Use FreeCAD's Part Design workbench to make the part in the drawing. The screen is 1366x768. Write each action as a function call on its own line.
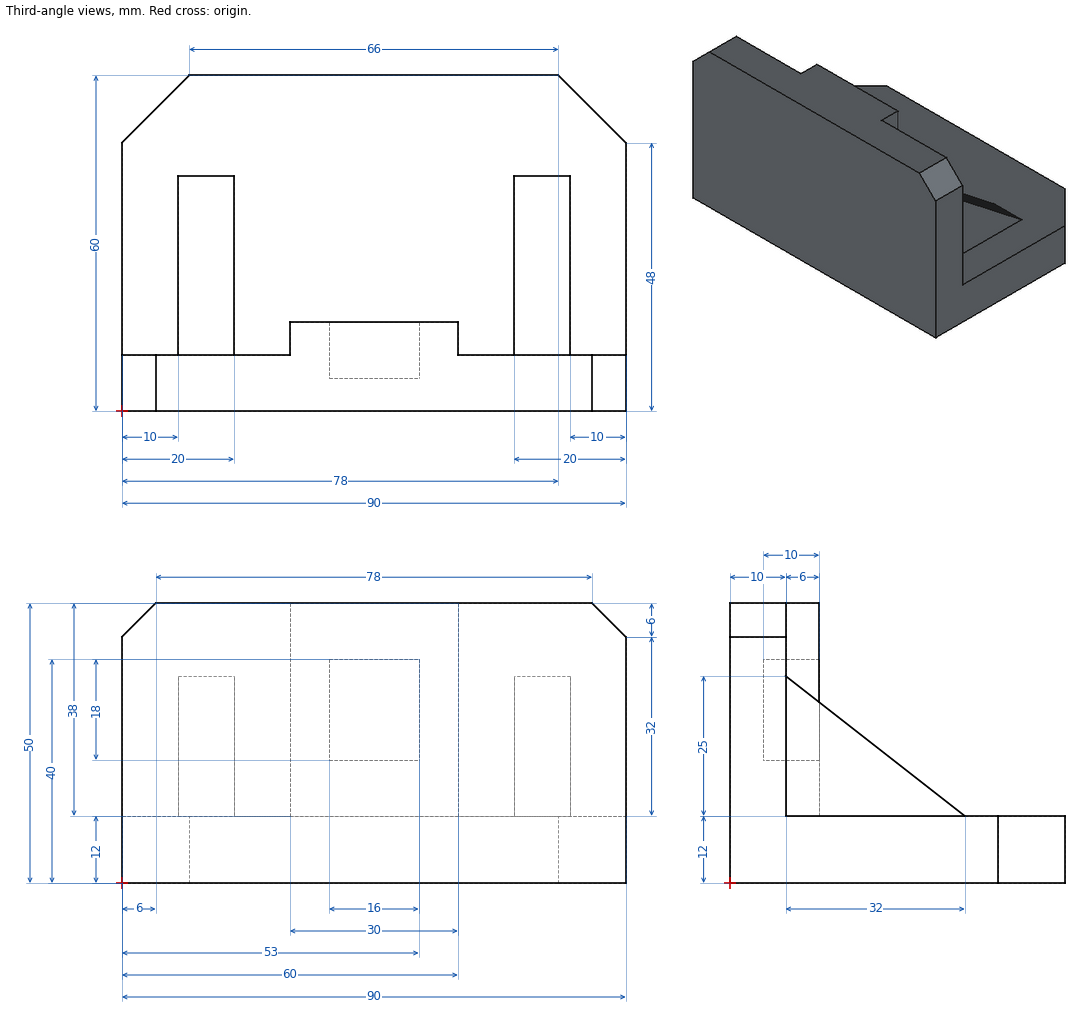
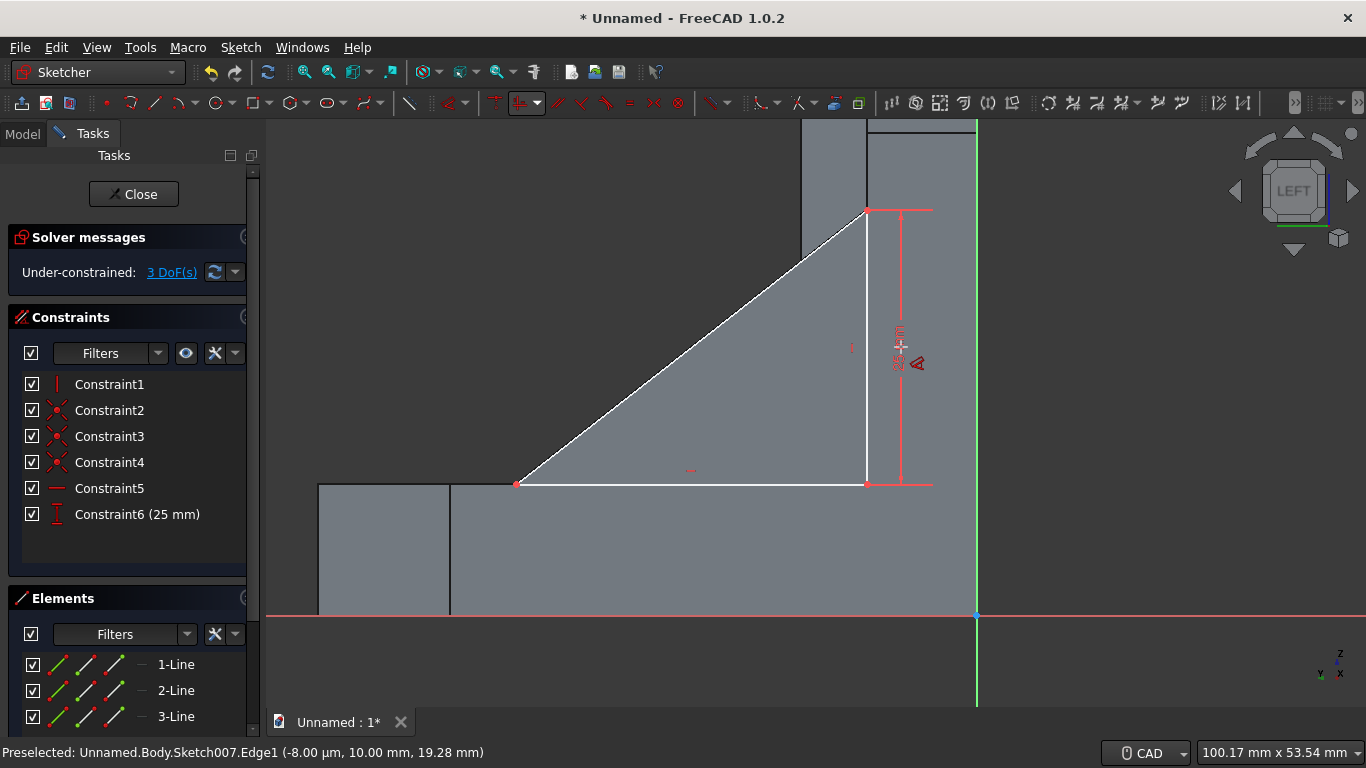
click(621, 485)
click(692, 519)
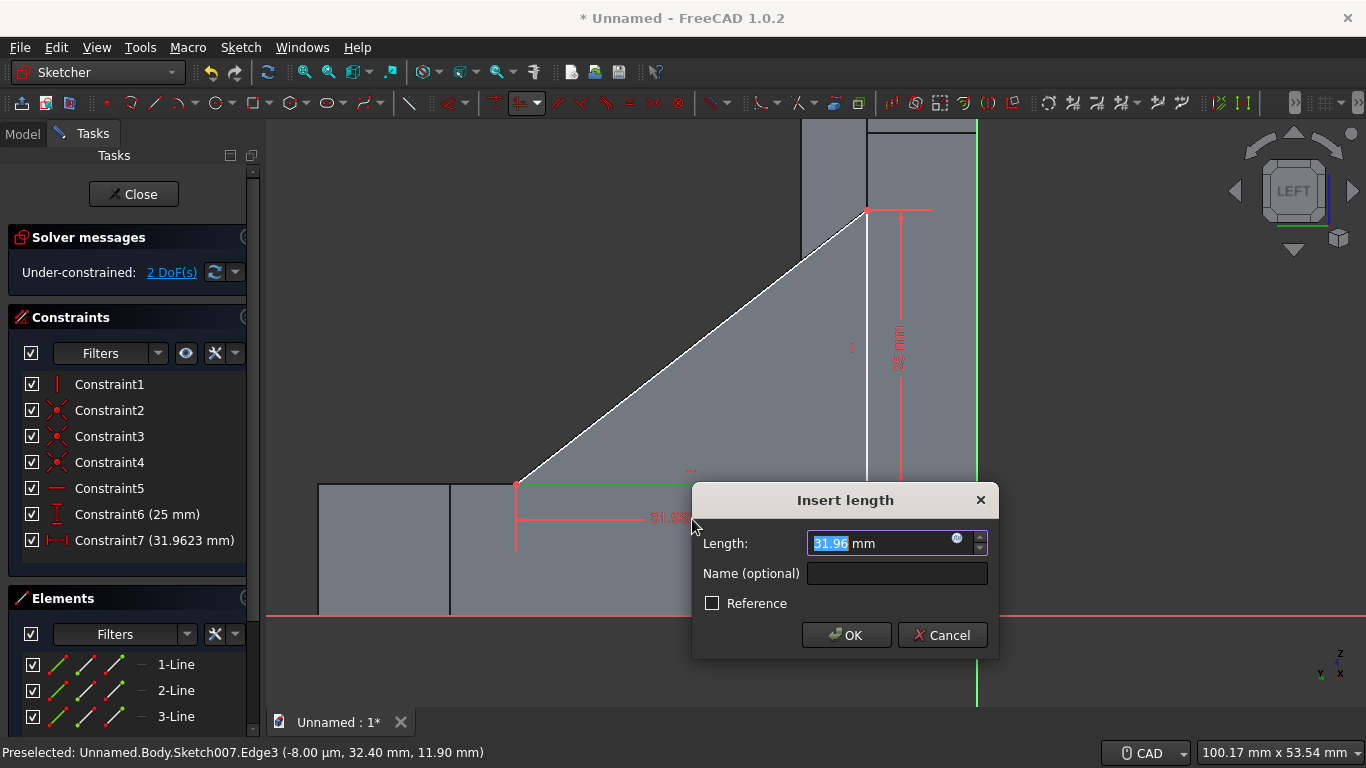
text(32)
key(Return)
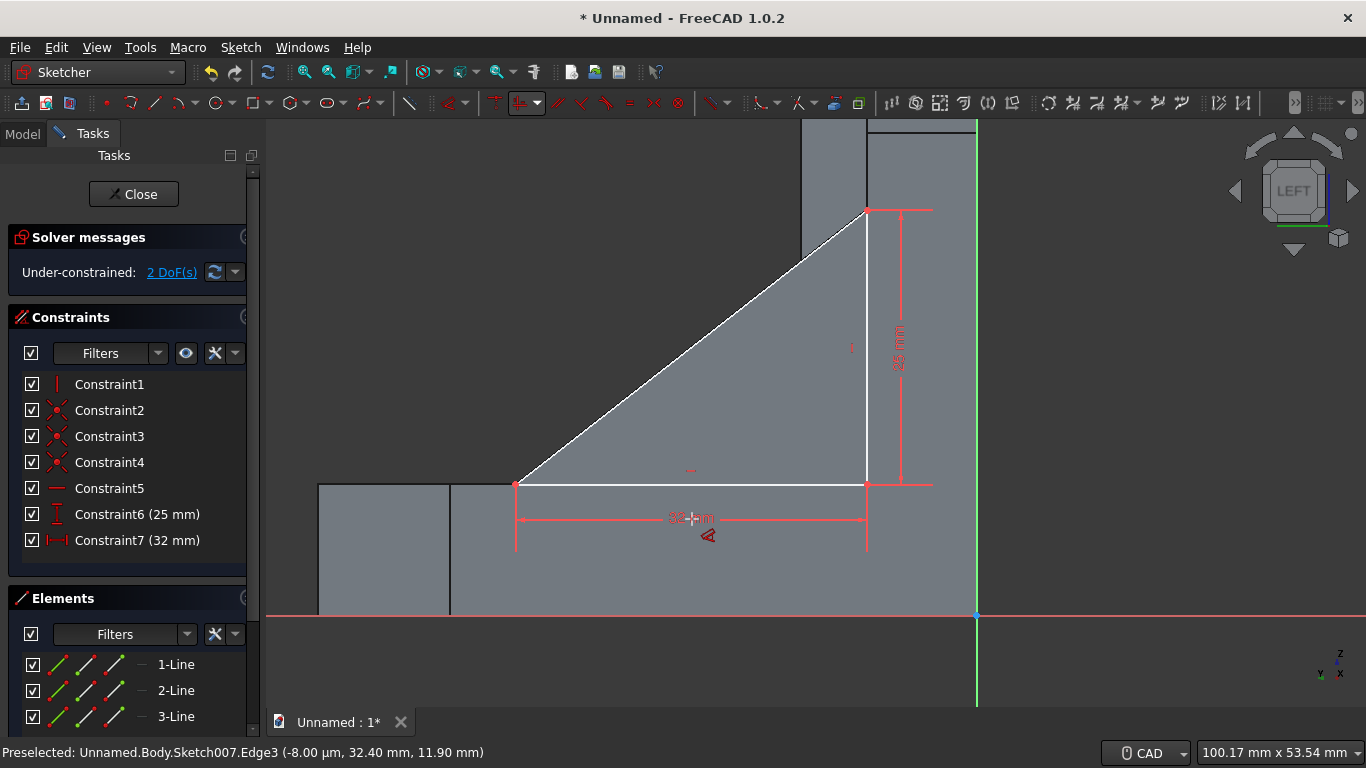
click(867, 485)
click(922, 650)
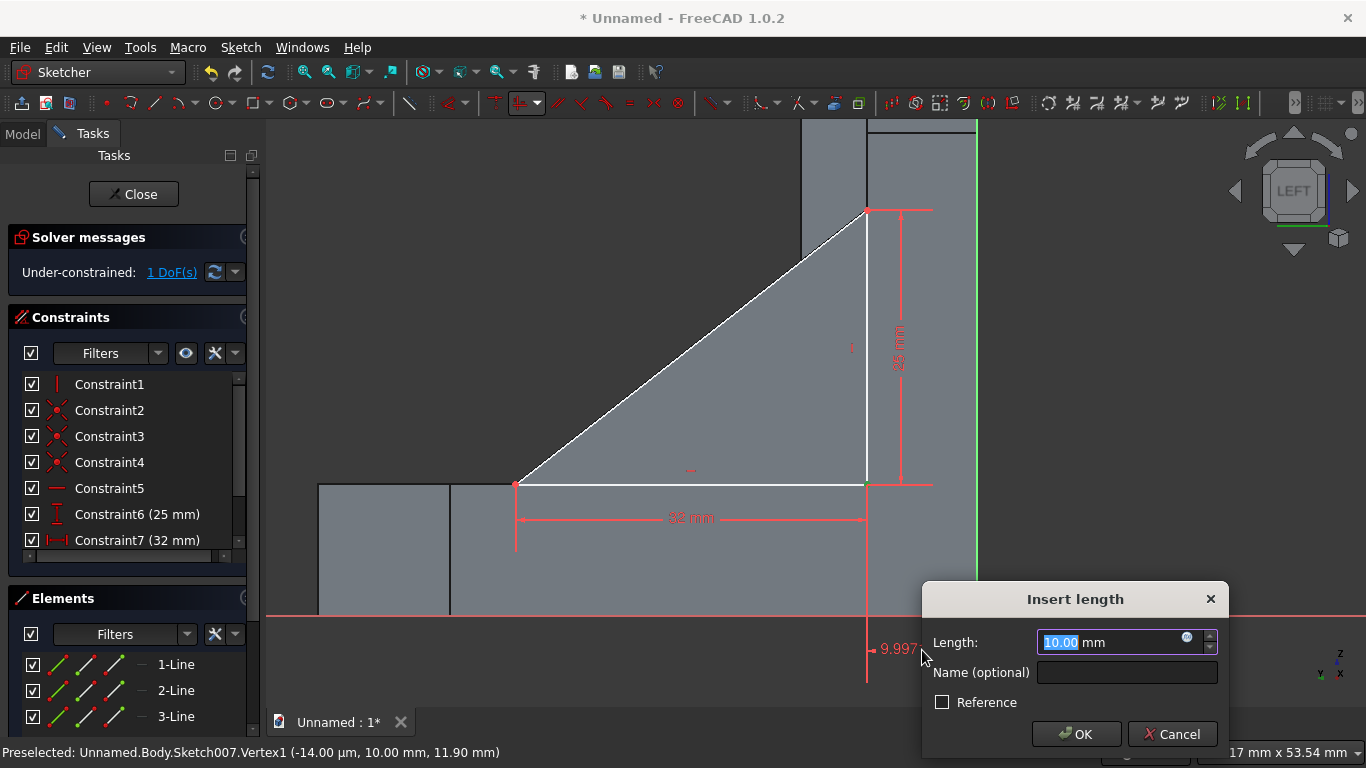
text(10)
key(Return)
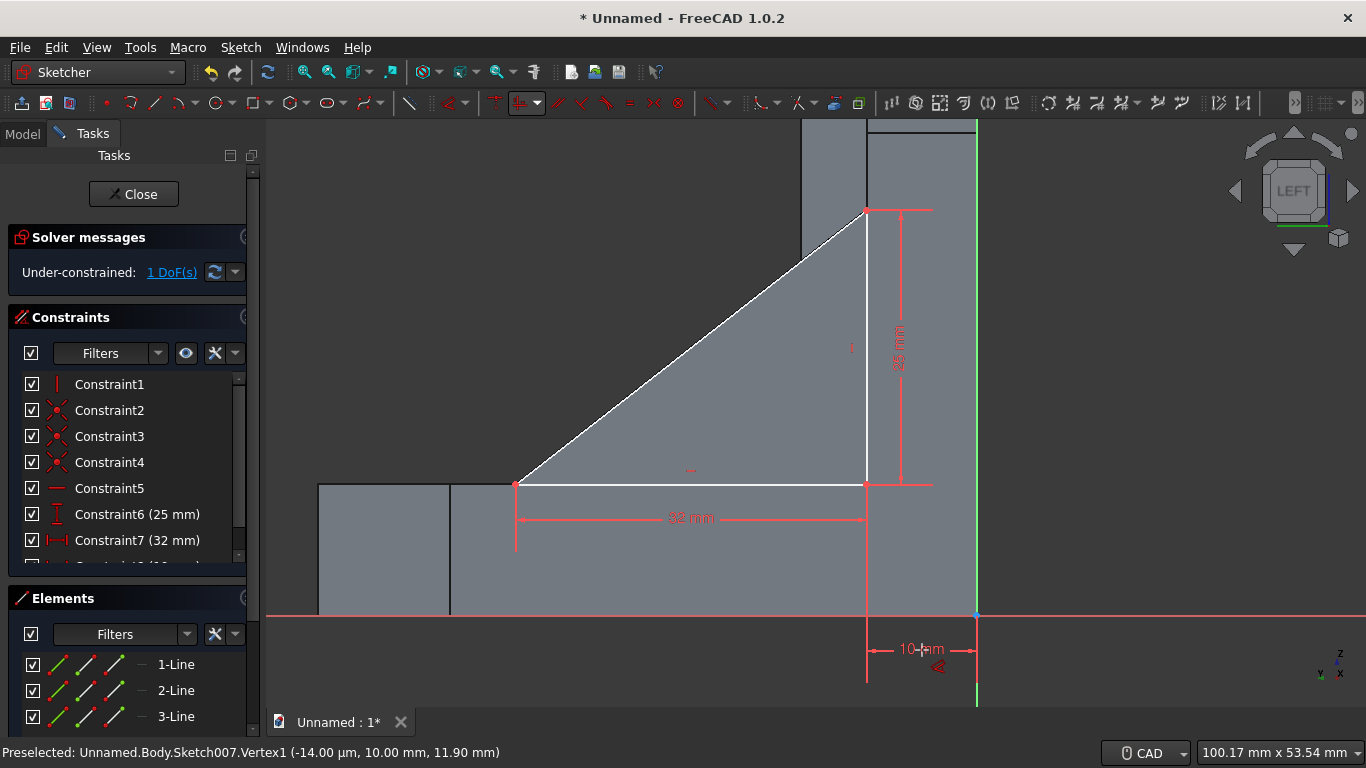
click(867, 485)
click(1011, 550)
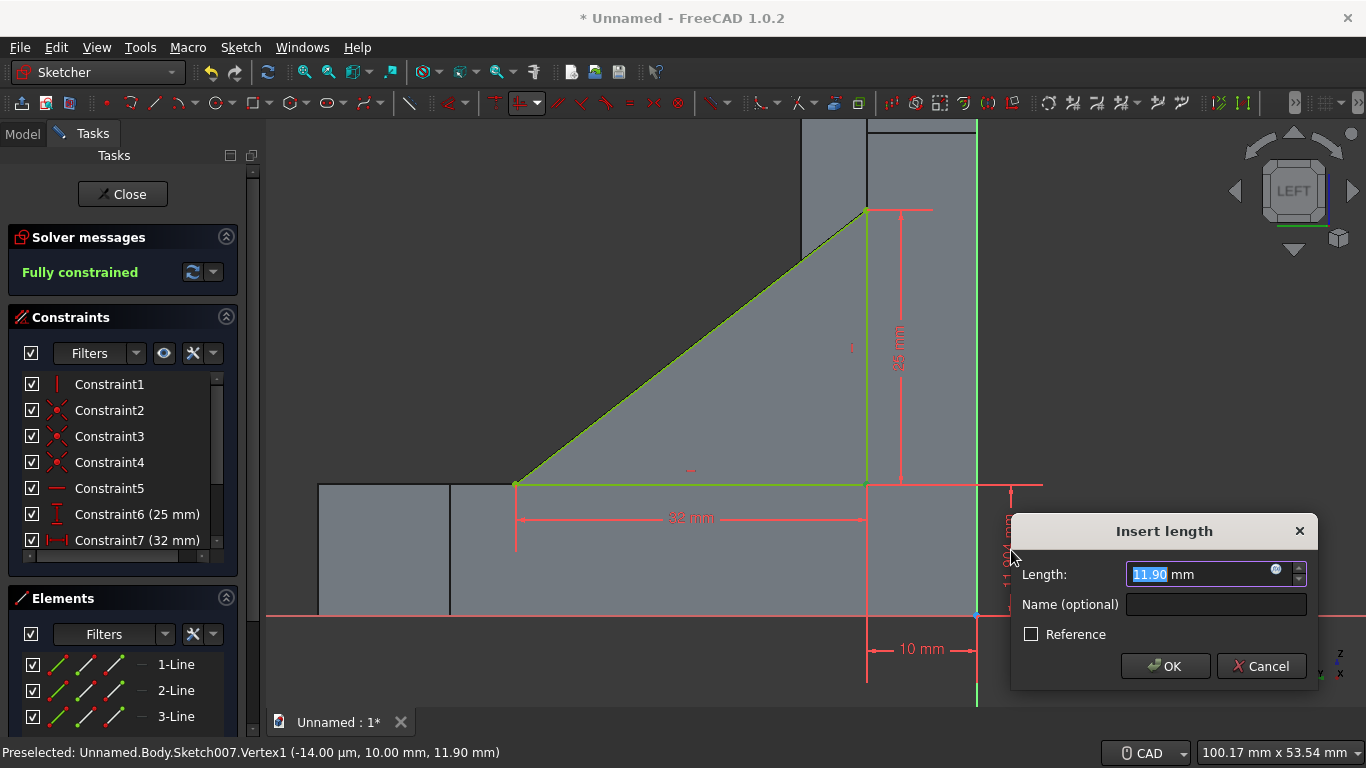
text(12)
key(Return)
key(Escape)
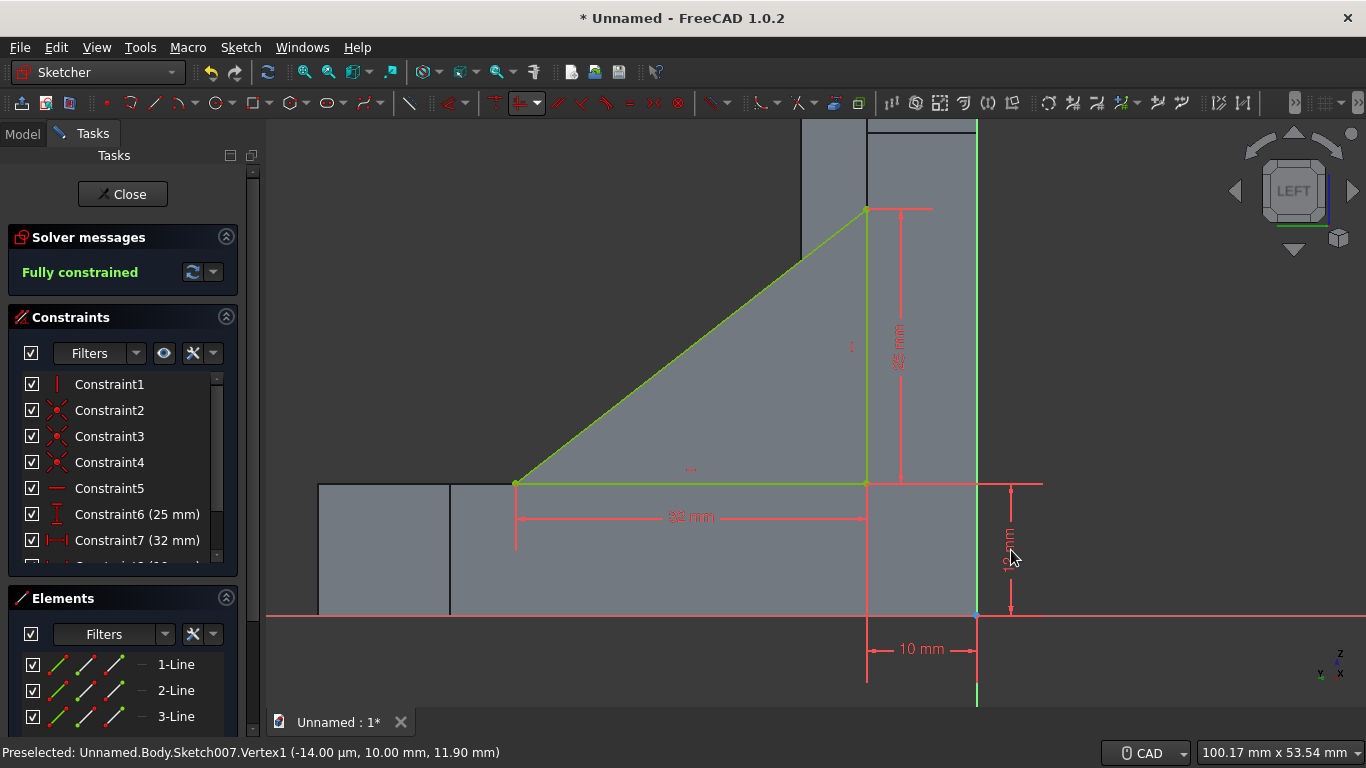
click(123, 194)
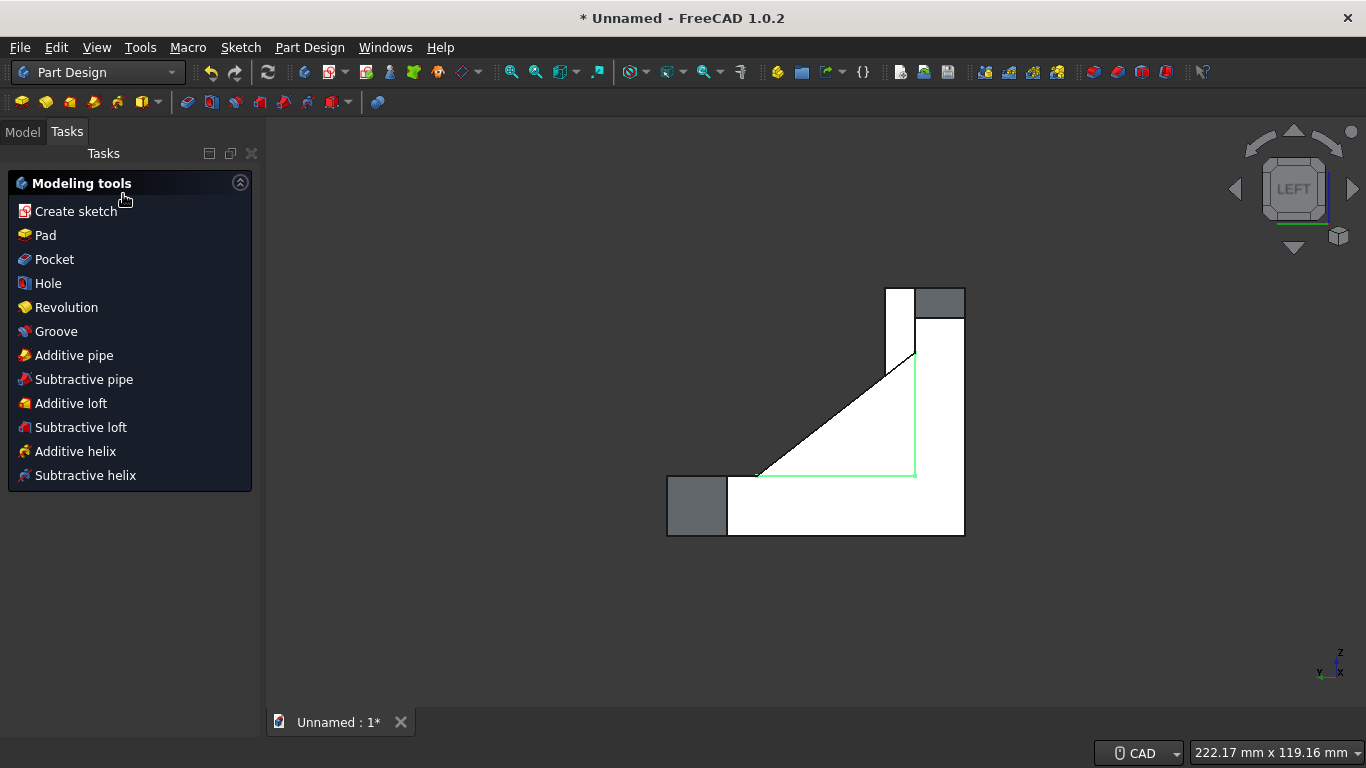
click(188, 102)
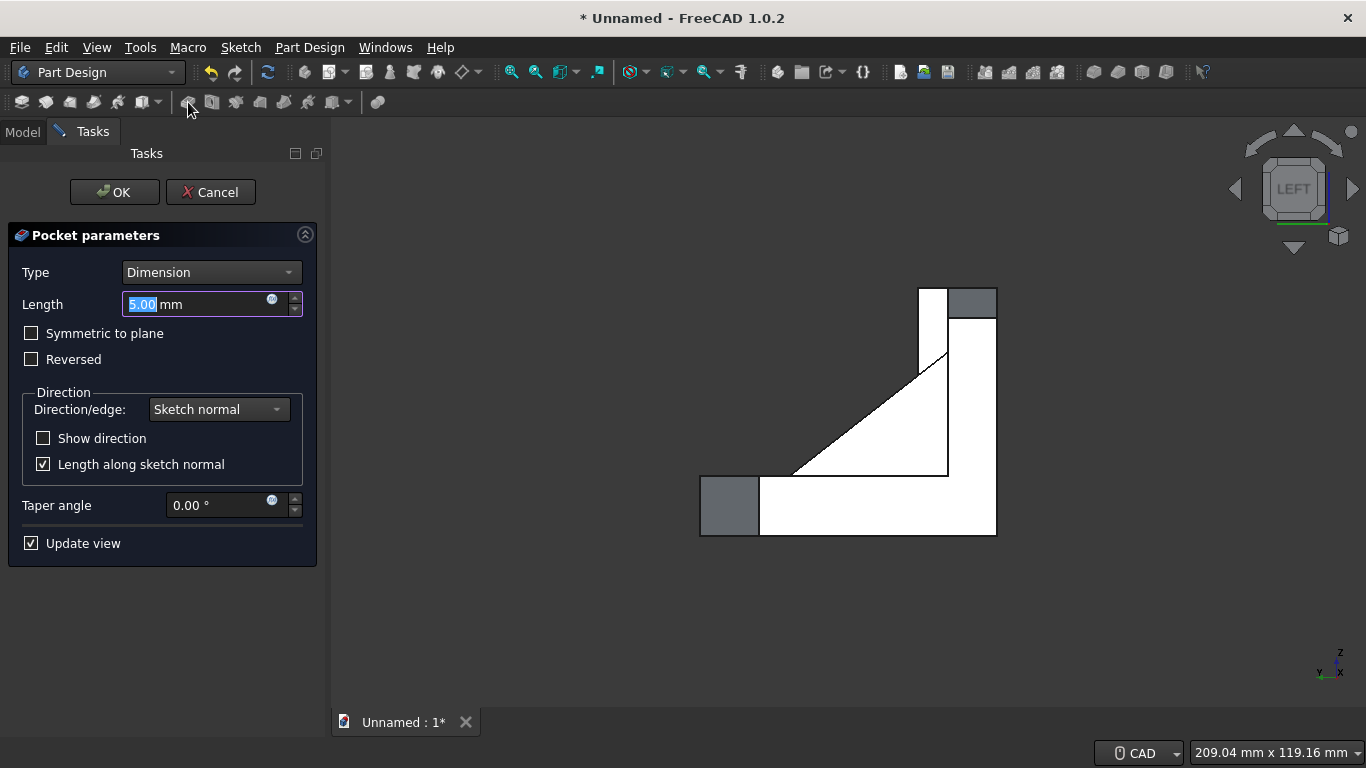
text(10)
key(Tab)